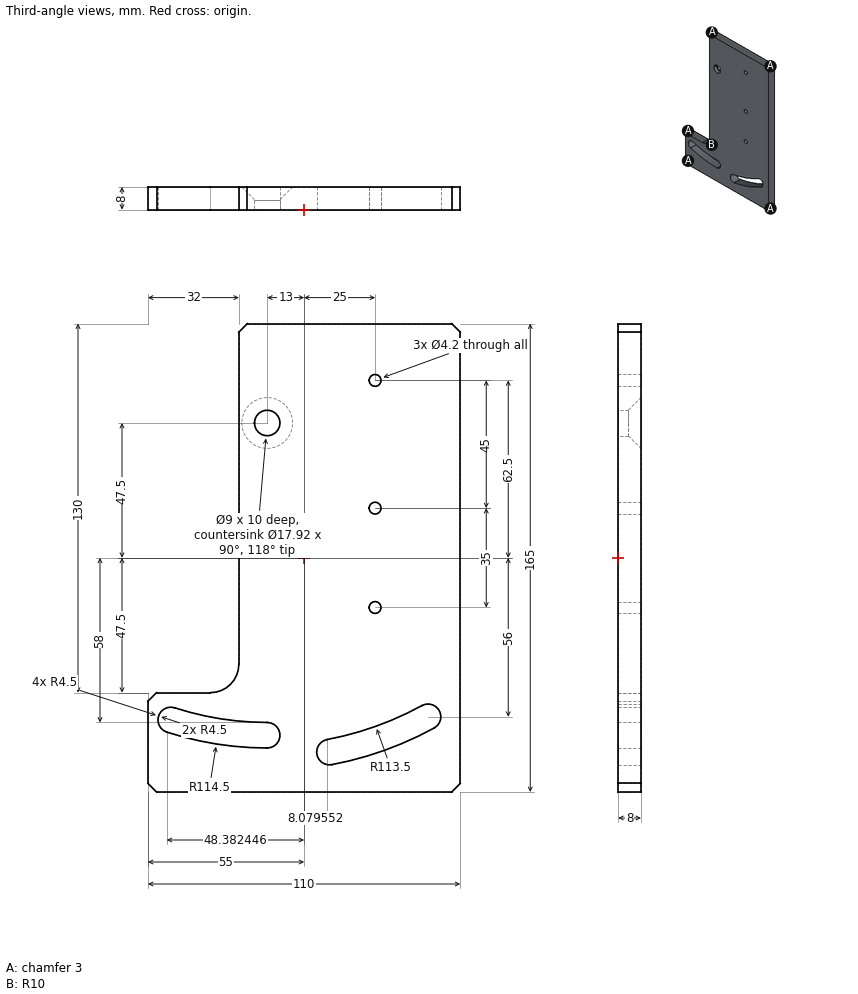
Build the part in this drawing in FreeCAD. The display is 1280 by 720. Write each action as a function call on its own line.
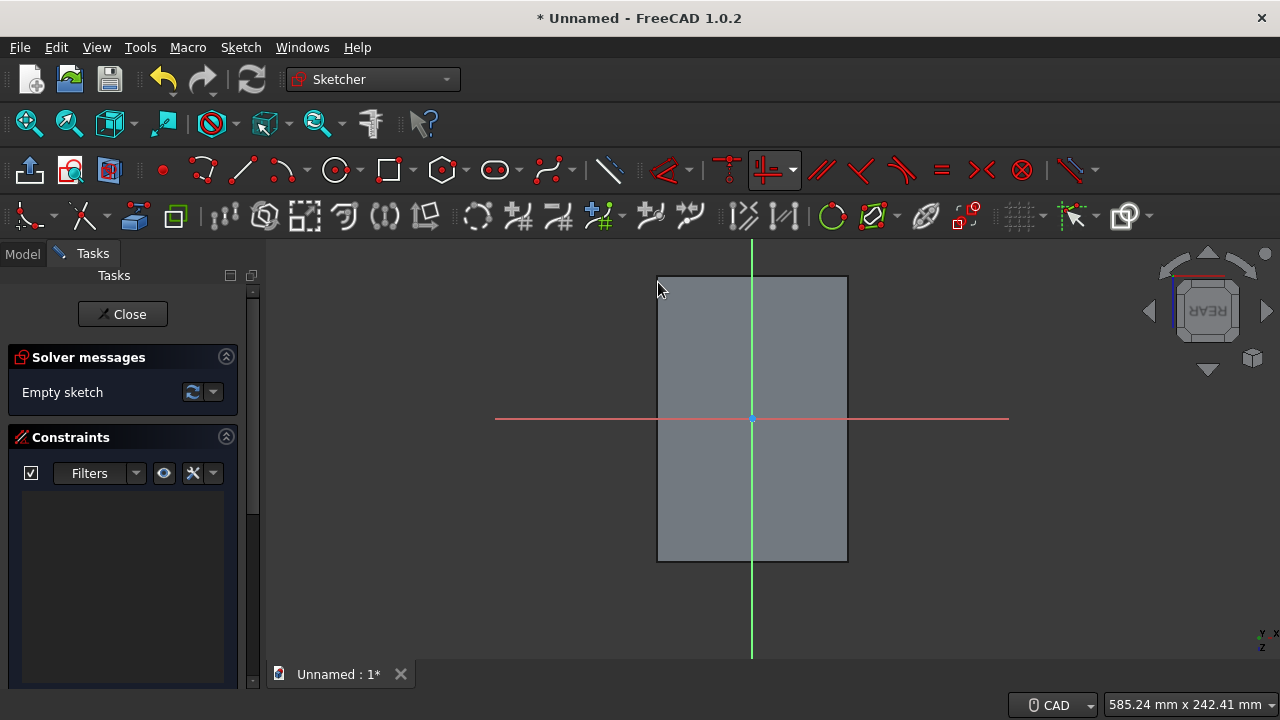
click(390, 170)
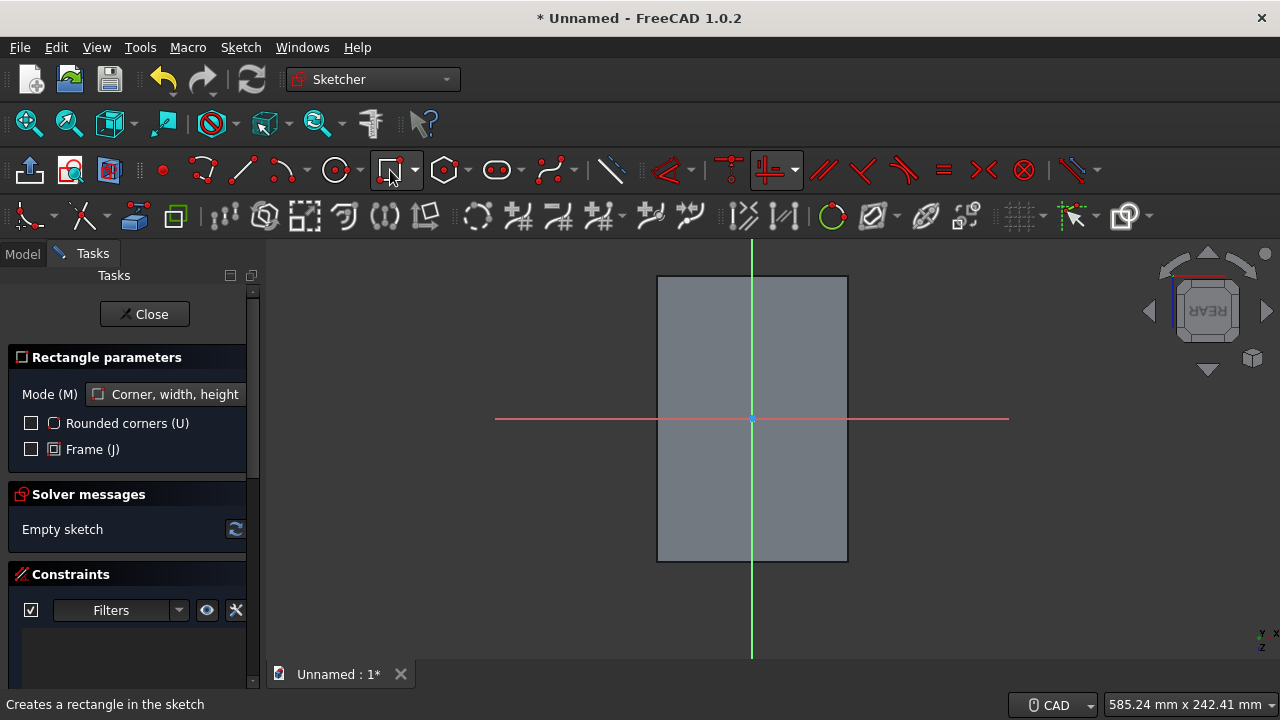
click(657, 336)
click(712, 562)
key(Escape)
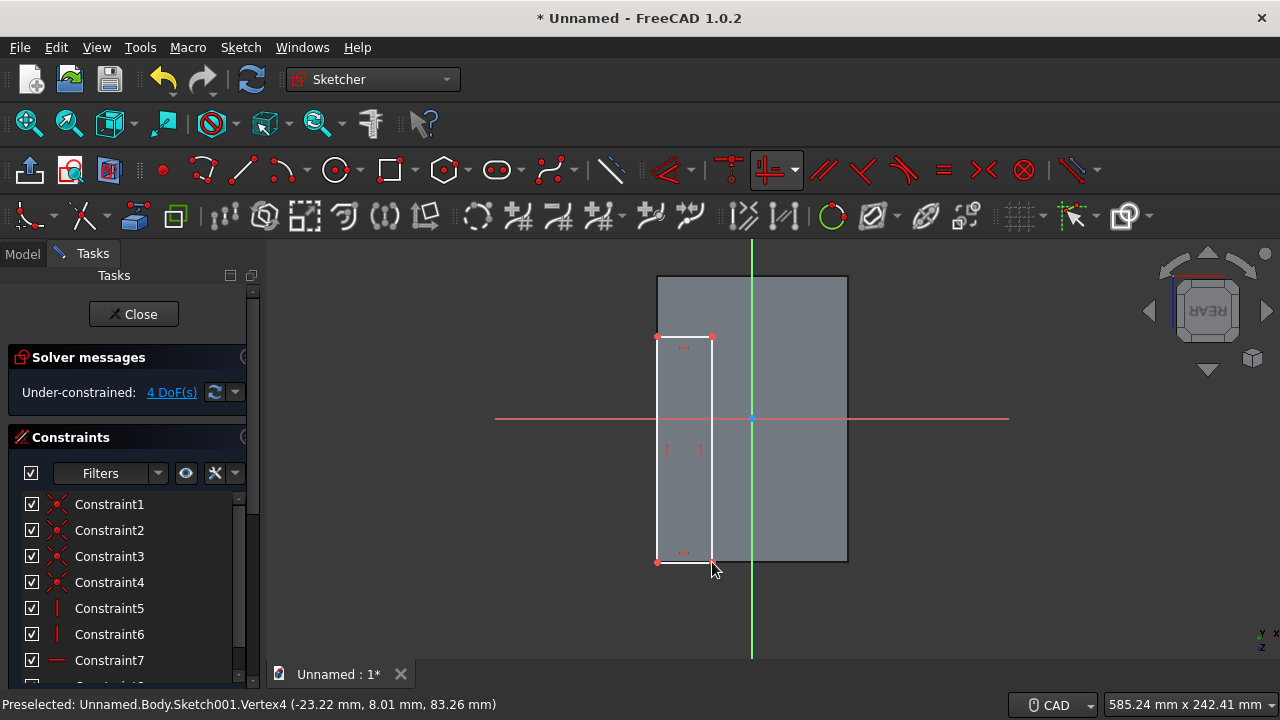
click(666, 170)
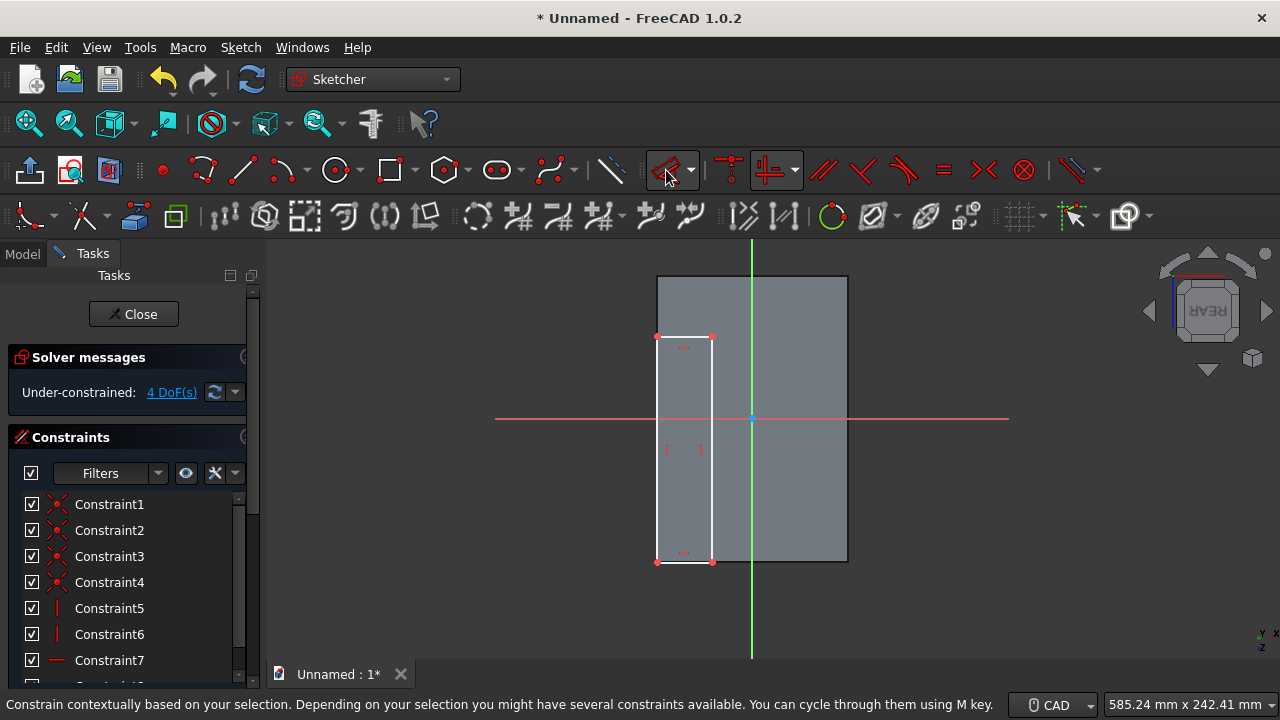
click(673, 563)
click(684, 597)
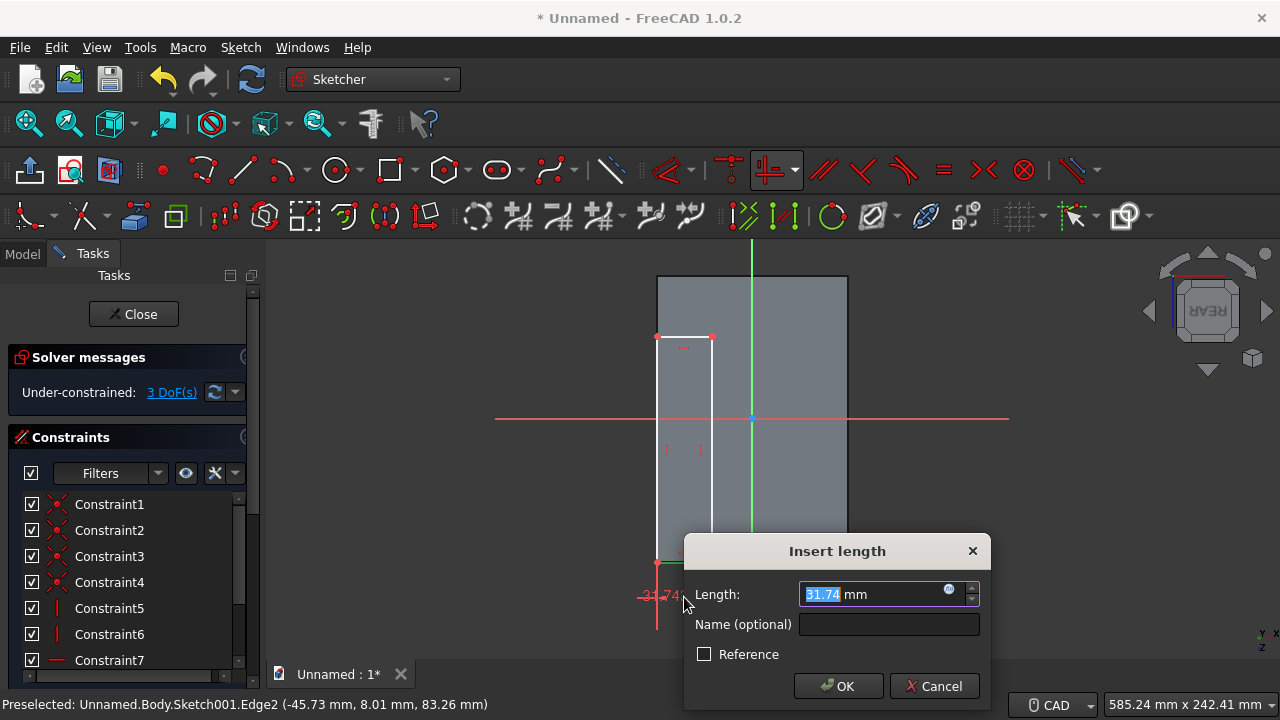
text(32)
key(Return)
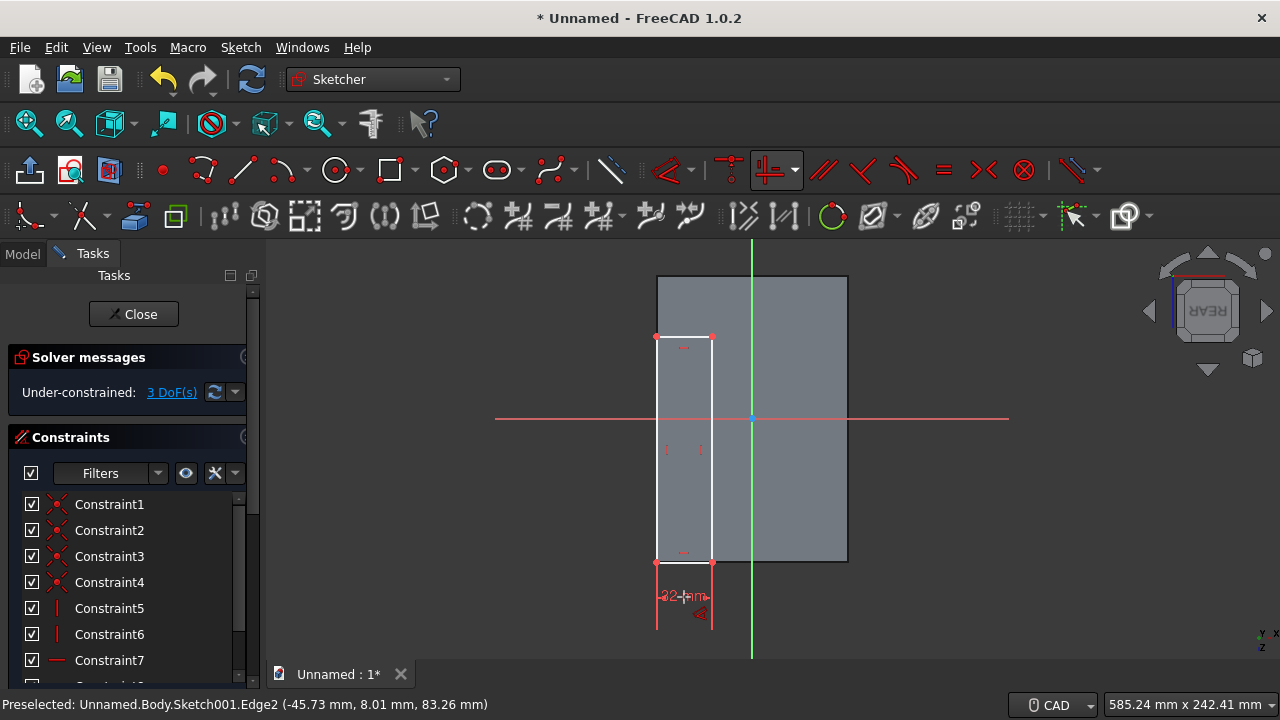
click(657, 405)
click(623, 450)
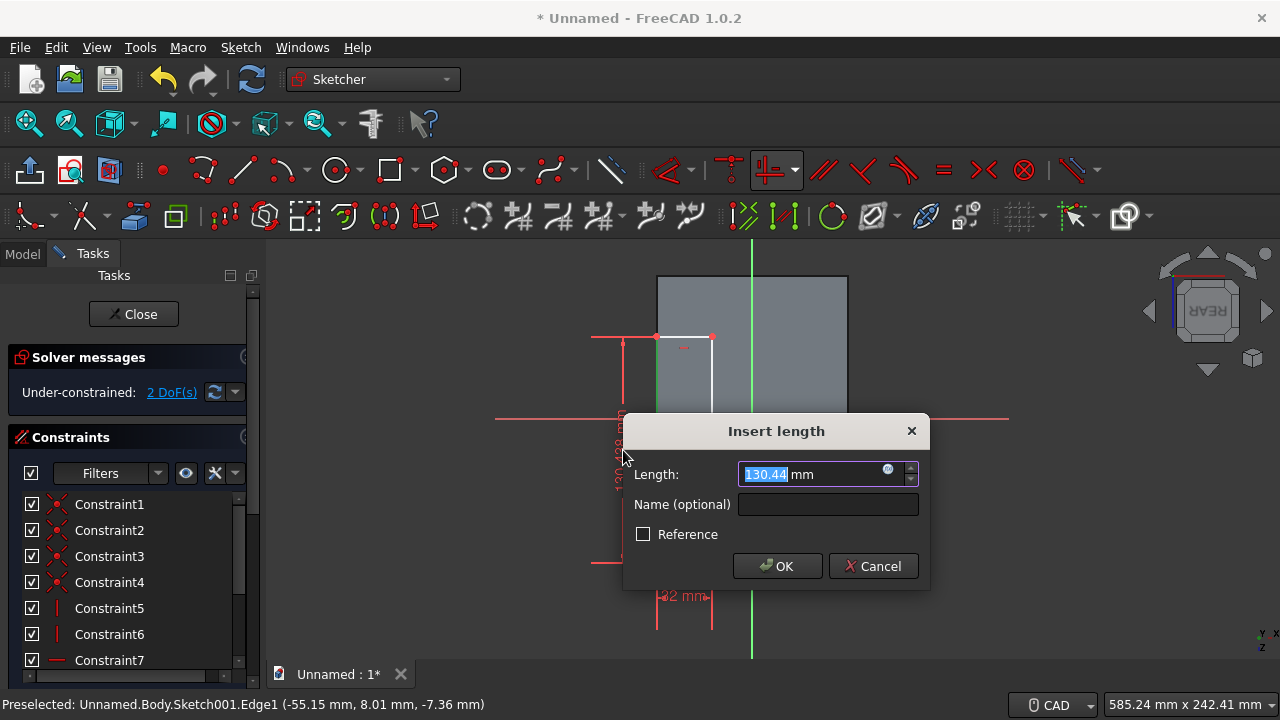
text(130)
key(Return)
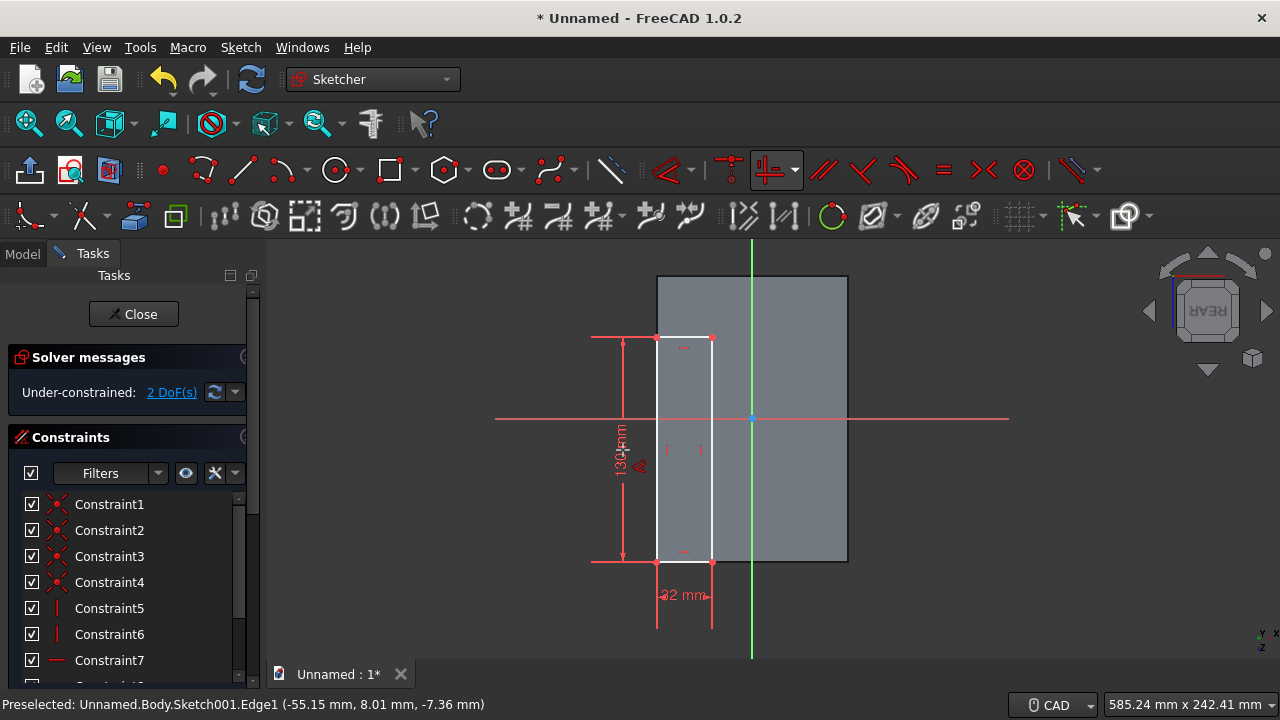
click(657, 337)
click(704, 303)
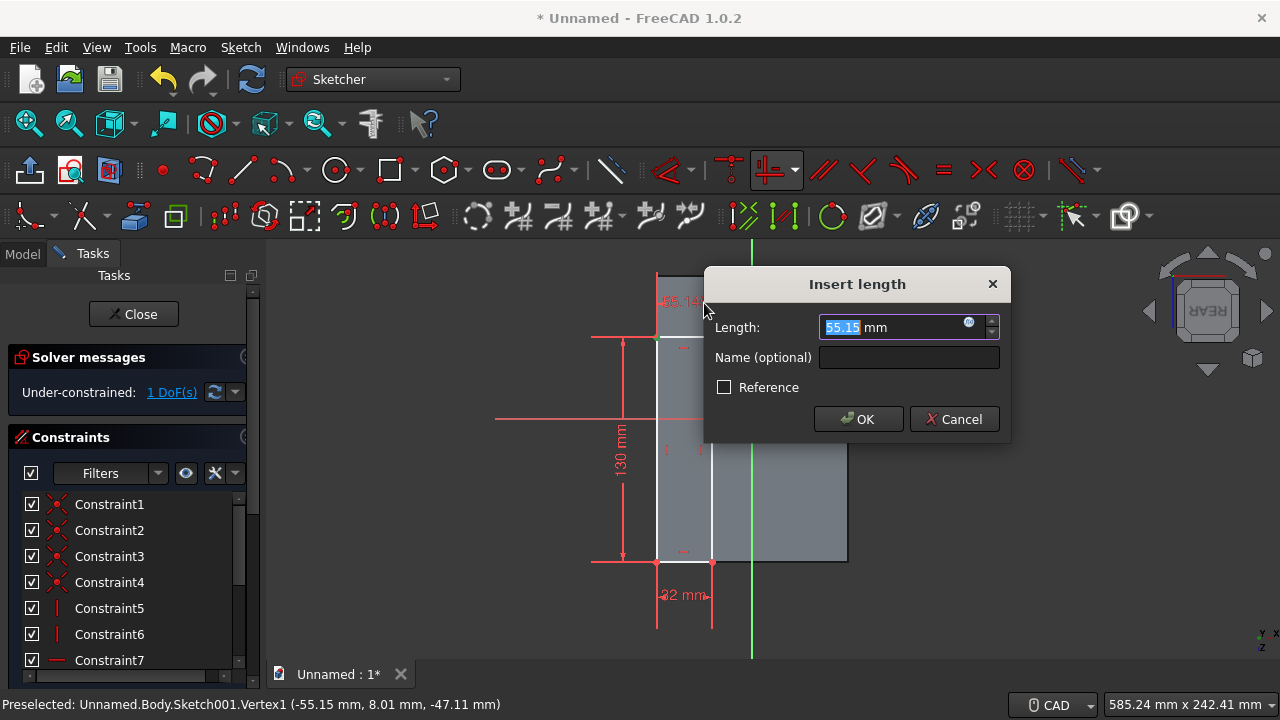
text(55)
key(Return)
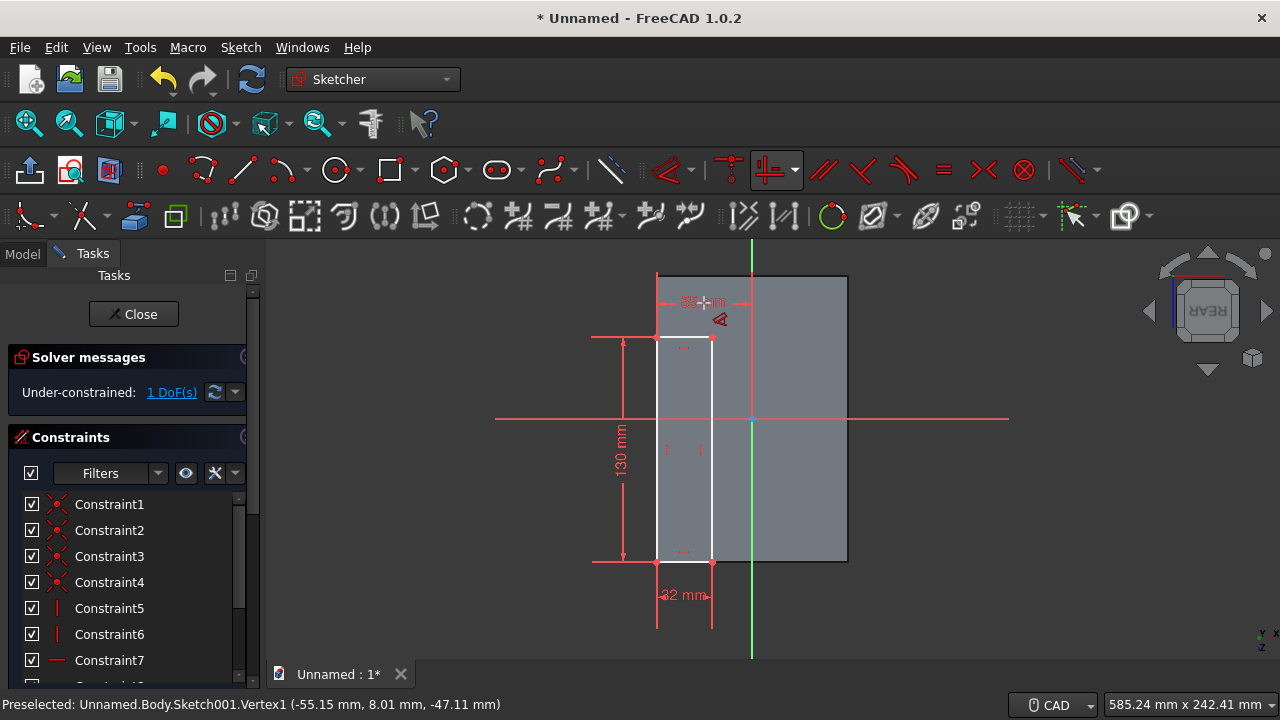
click(657, 337)
click(786, 378)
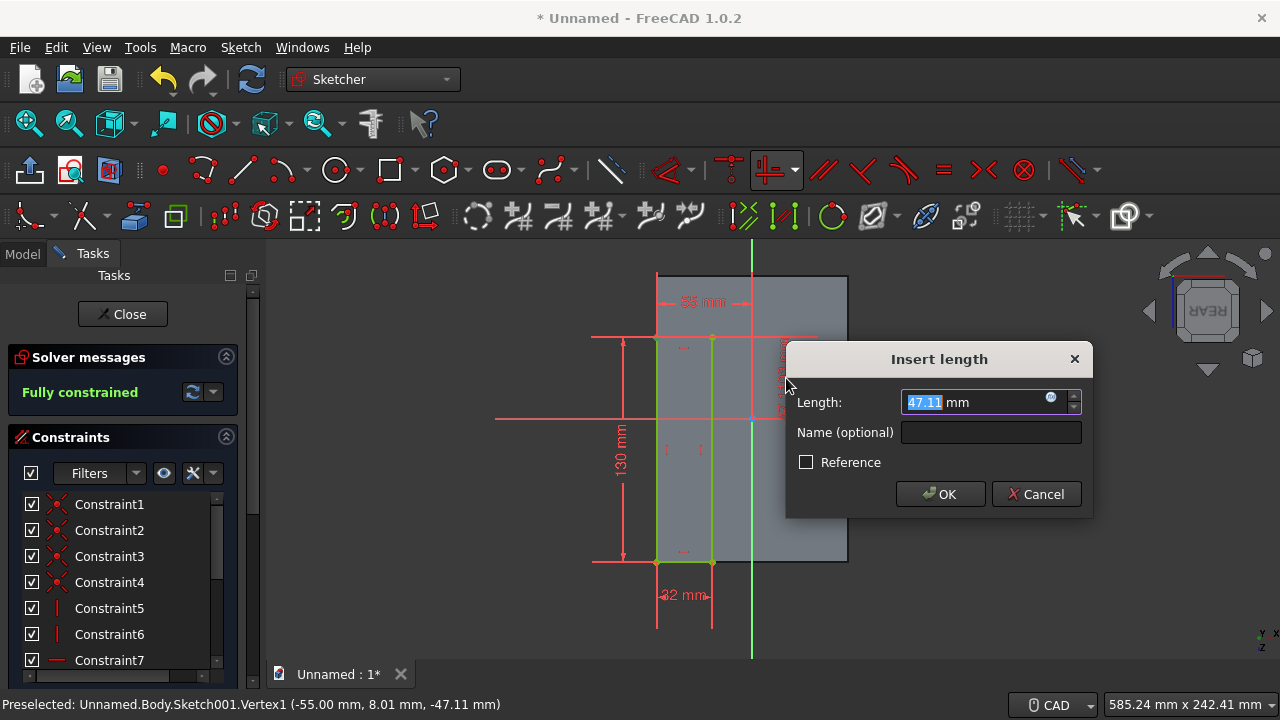
text(47.5)
key(Return)
key(Escape)